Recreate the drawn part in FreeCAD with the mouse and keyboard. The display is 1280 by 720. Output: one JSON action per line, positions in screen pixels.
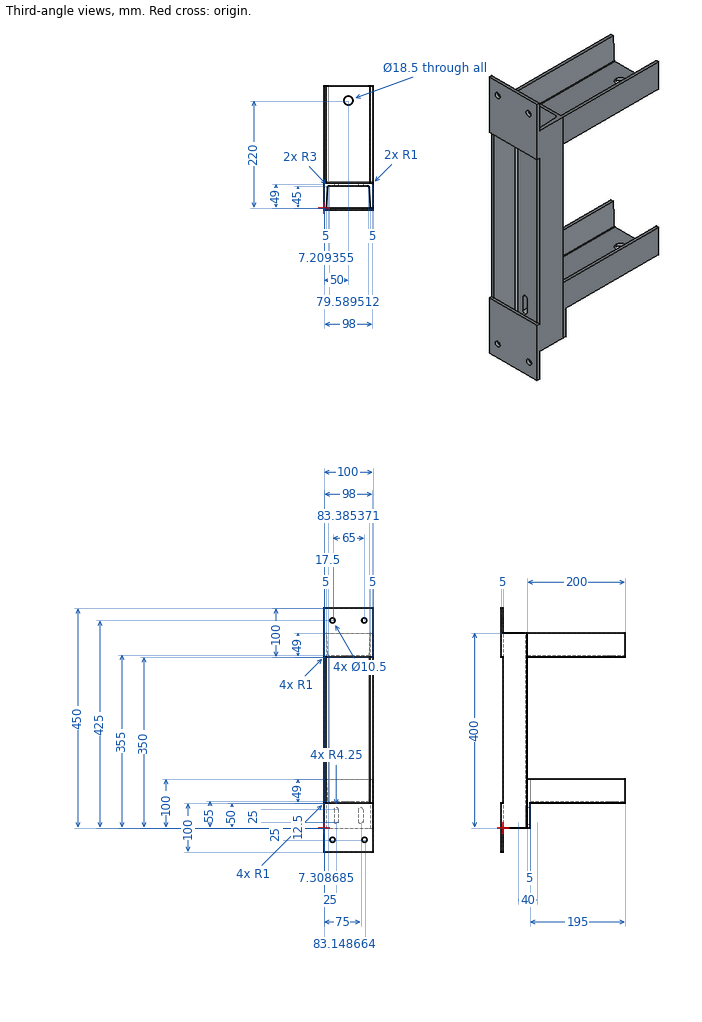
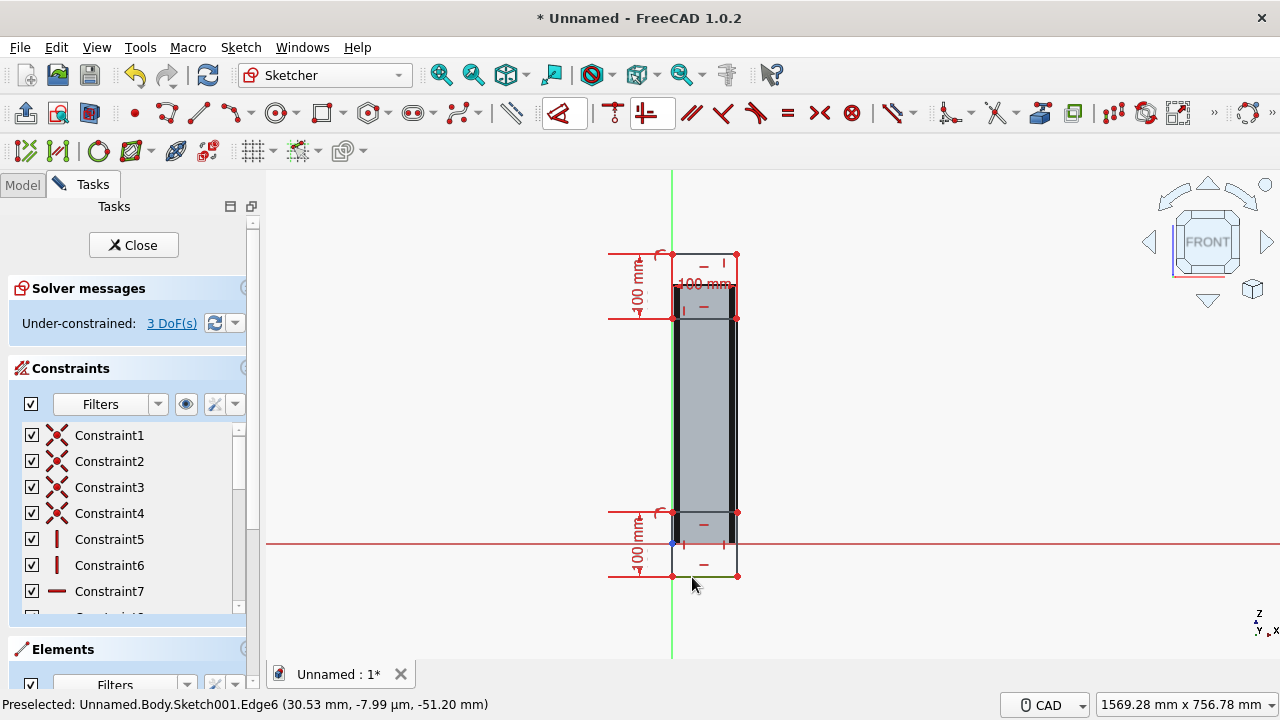
{"action": "key", "text": "l"}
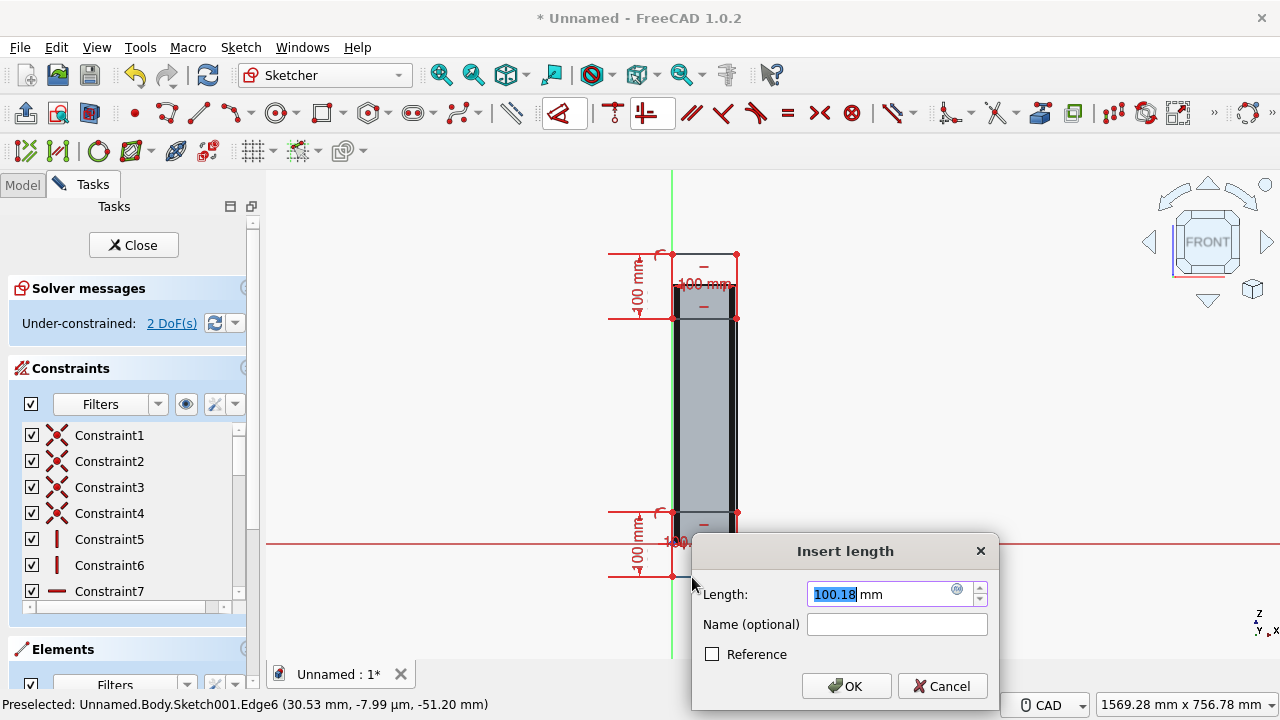
{"action": "type", "text": "100"}
{"action": "key", "text": "Return"}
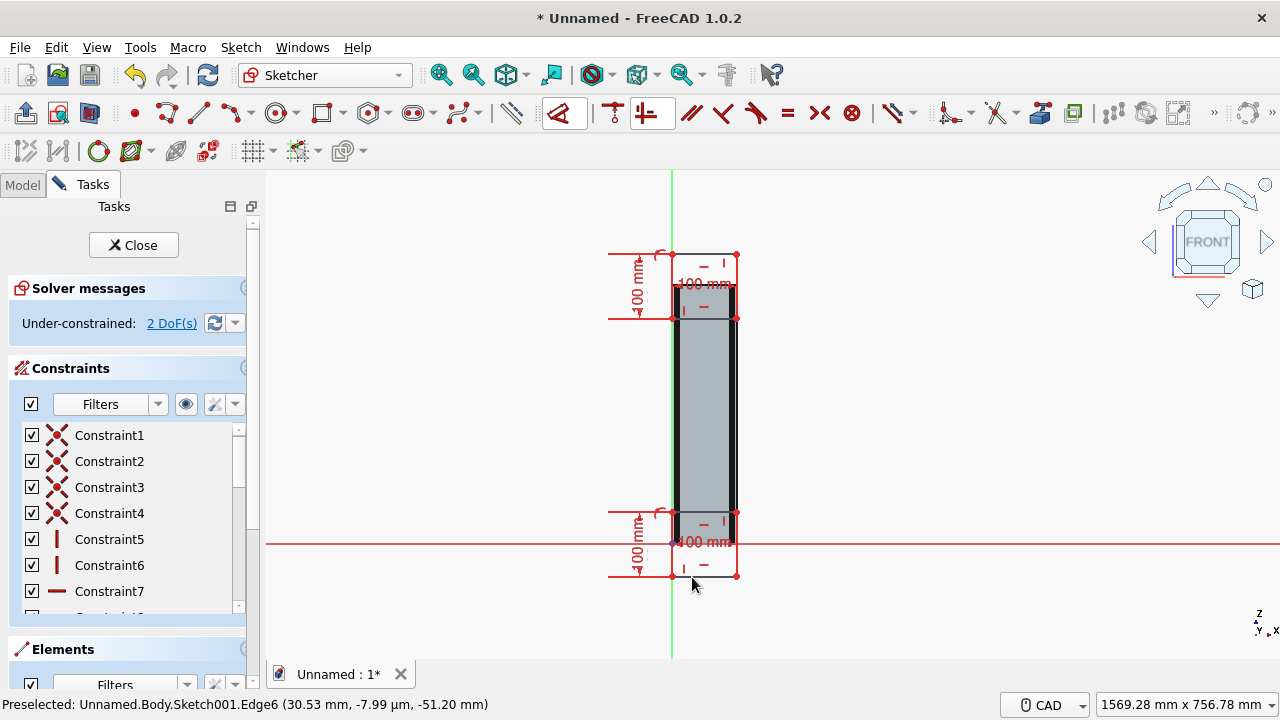
{"action": "scroll", "coordinate": [672, 512], "scroll_direction": "up", "scroll_amount": 2}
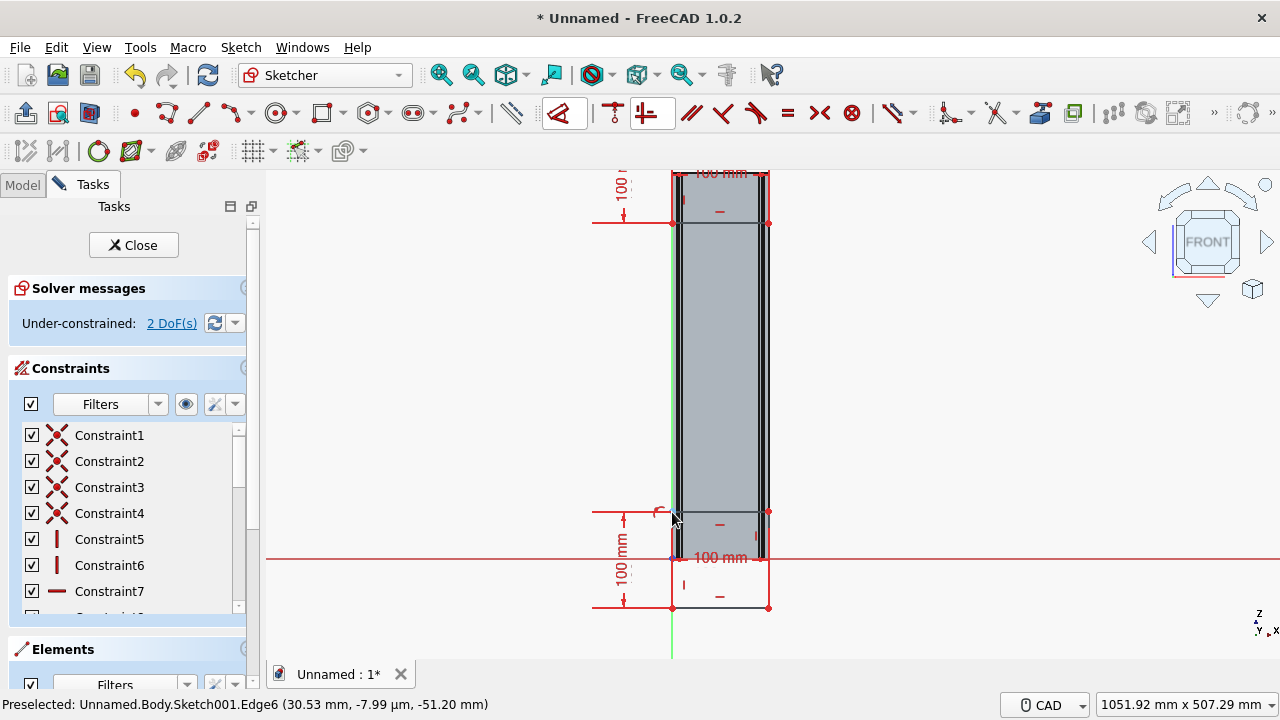
{"action": "left_click", "coordinate": [672, 512]}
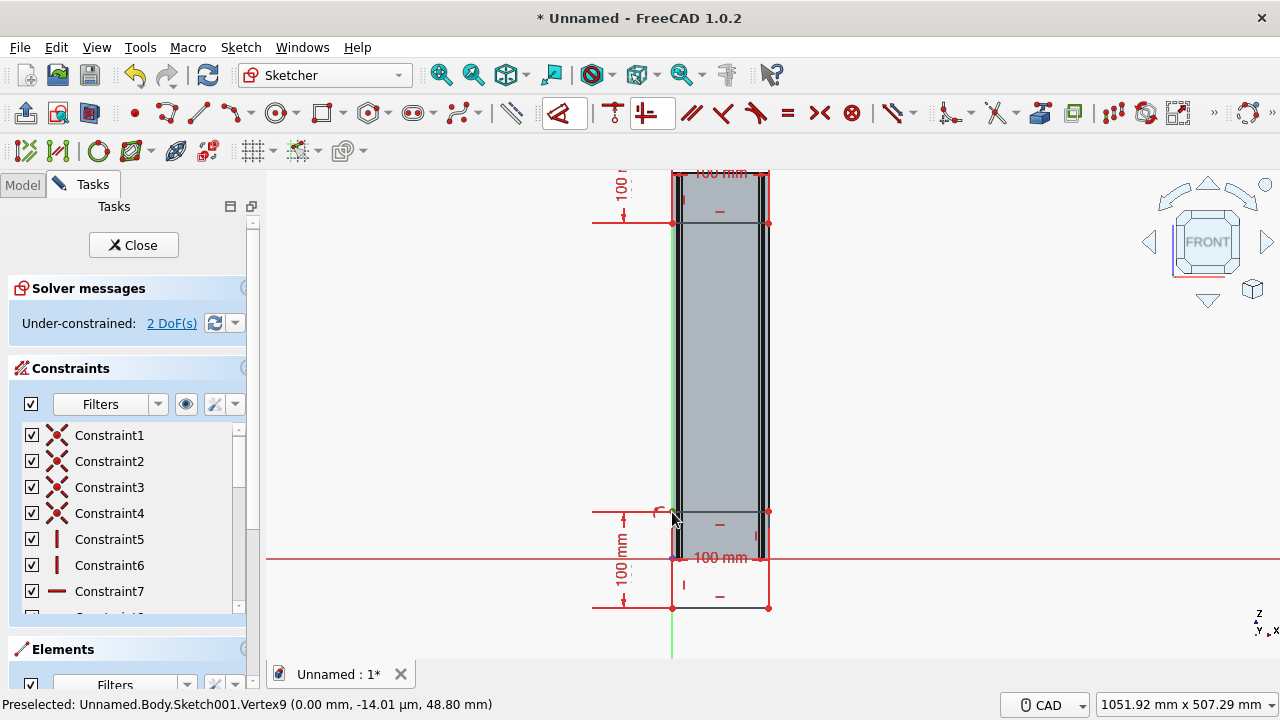
{"action": "left_click", "coordinate": [582, 114]}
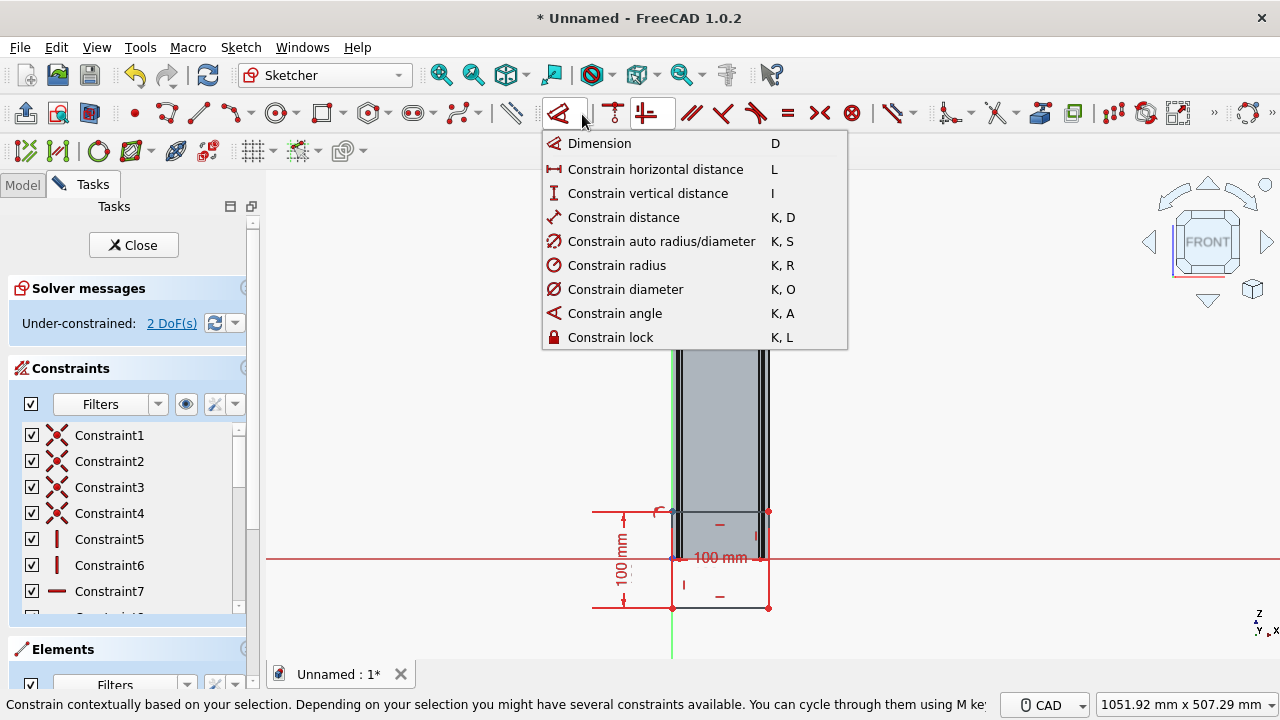
{"action": "left_click", "coordinate": [695, 193]}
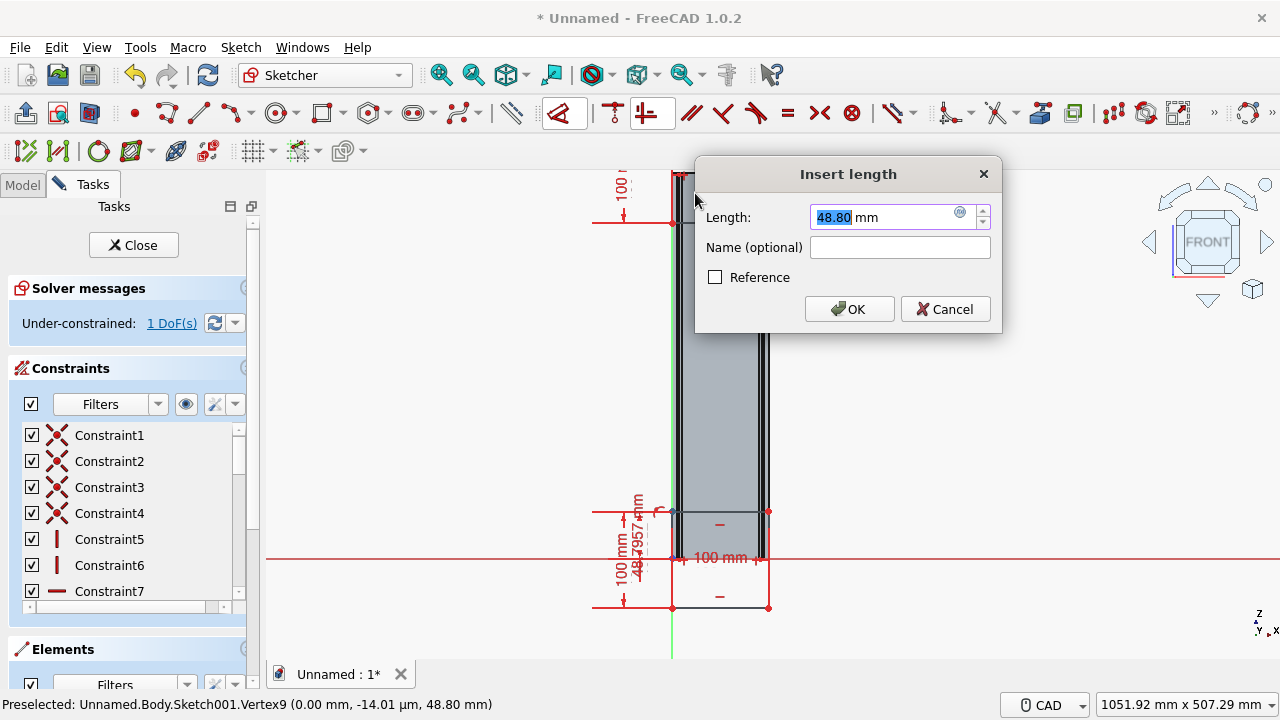
{"action": "type", "text": "50"}
{"action": "key", "text": "Return"}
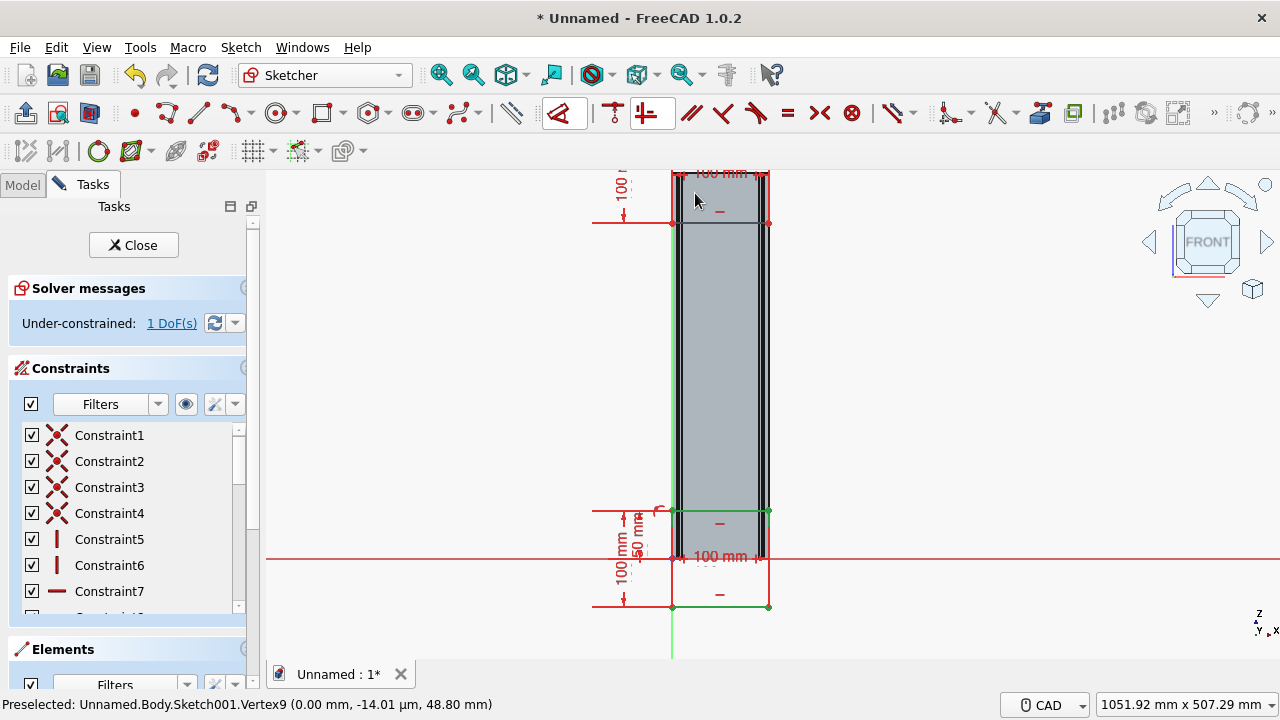
{"action": "scroll", "coordinate": [672, 513], "scroll_direction": "down", "scroll_amount": 2}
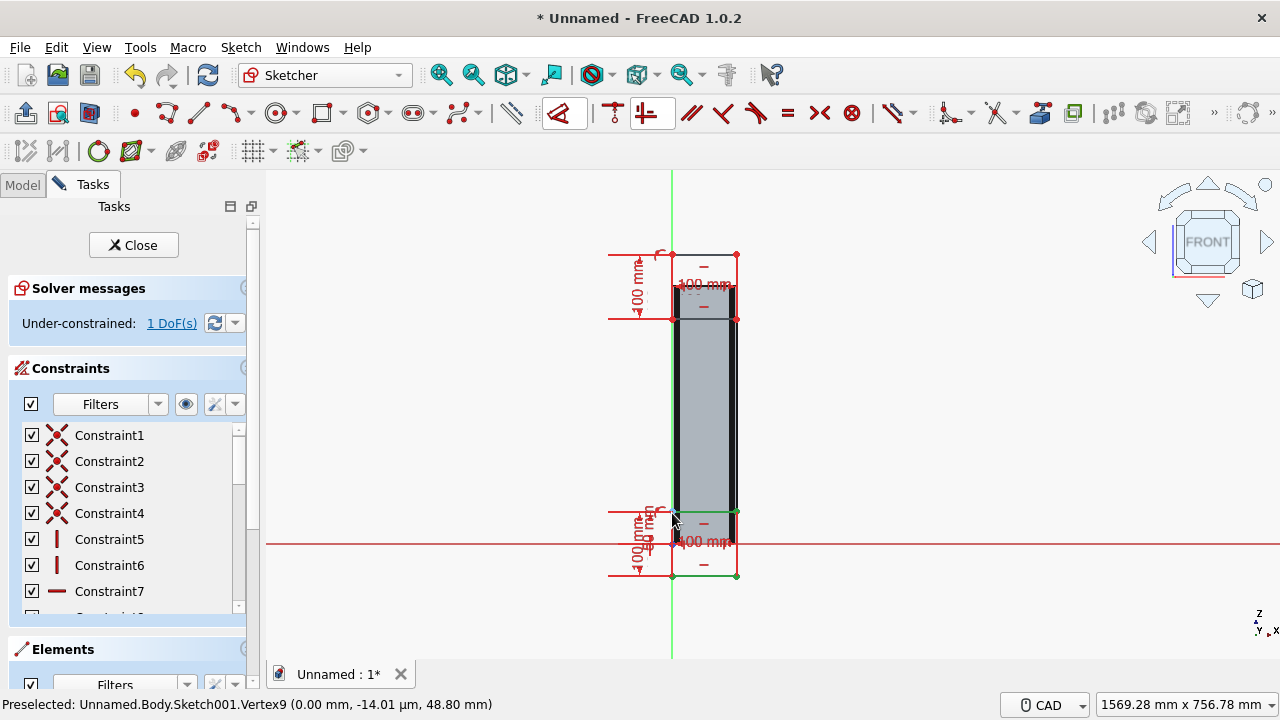
{"action": "left_click", "coordinate": [672, 255]}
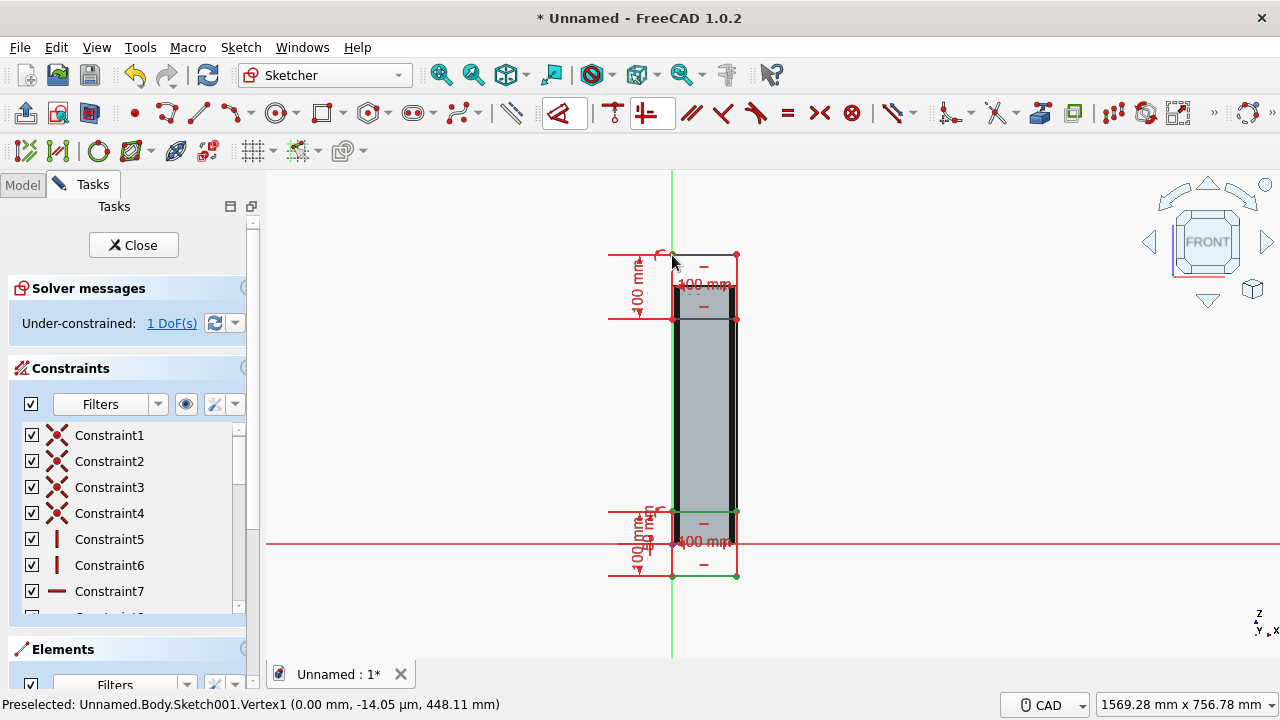
{"action": "key", "text": "i"}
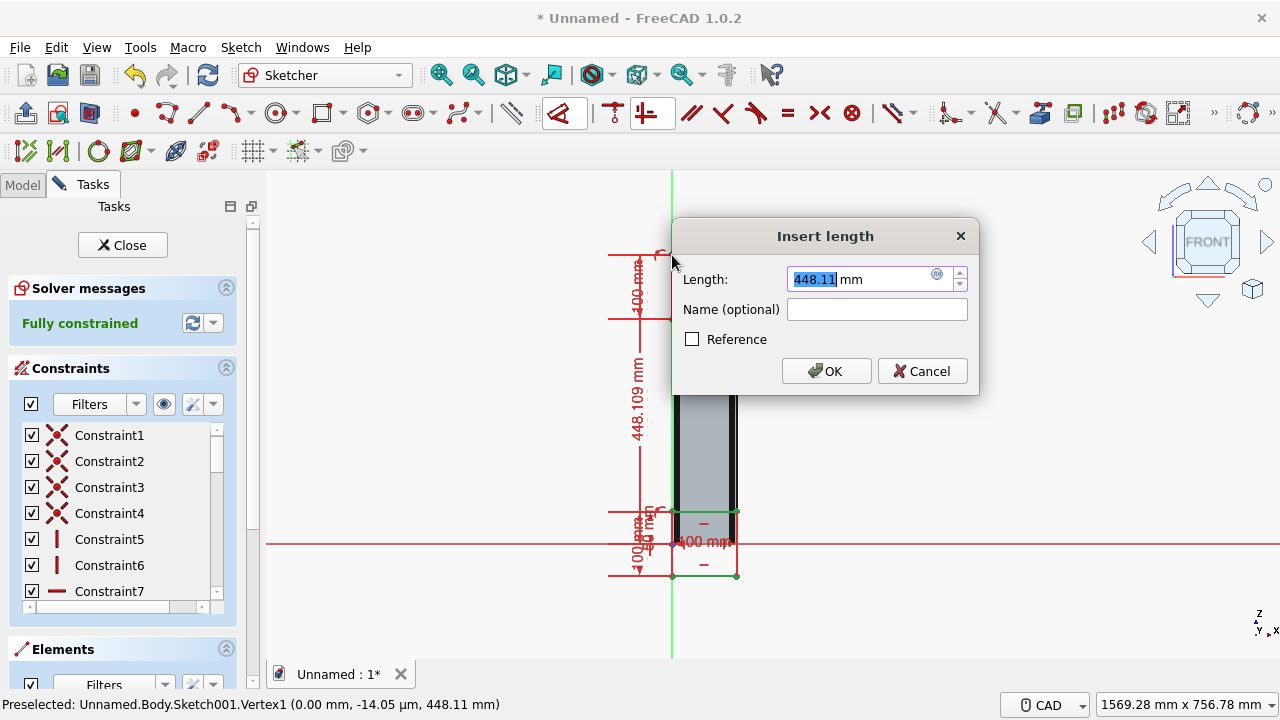
{"action": "type", "text": "450"}
{"action": "key", "text": "Return"}